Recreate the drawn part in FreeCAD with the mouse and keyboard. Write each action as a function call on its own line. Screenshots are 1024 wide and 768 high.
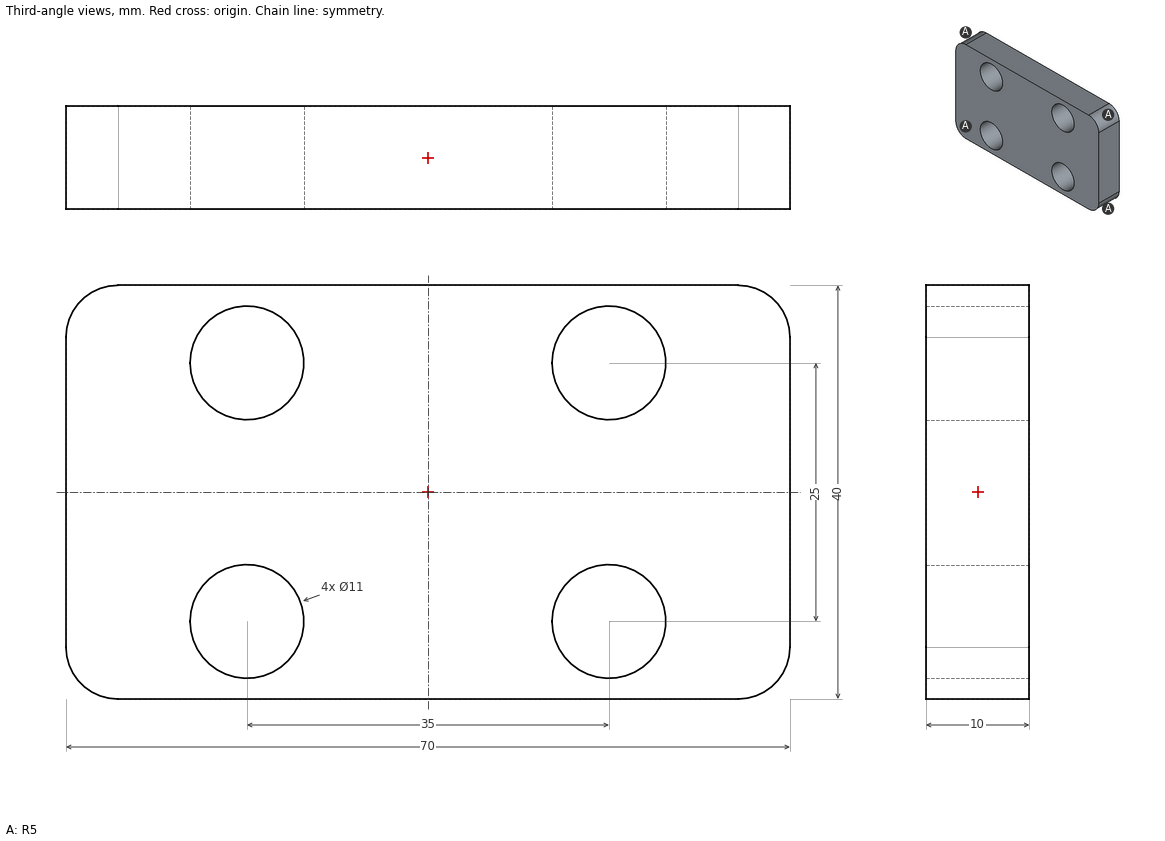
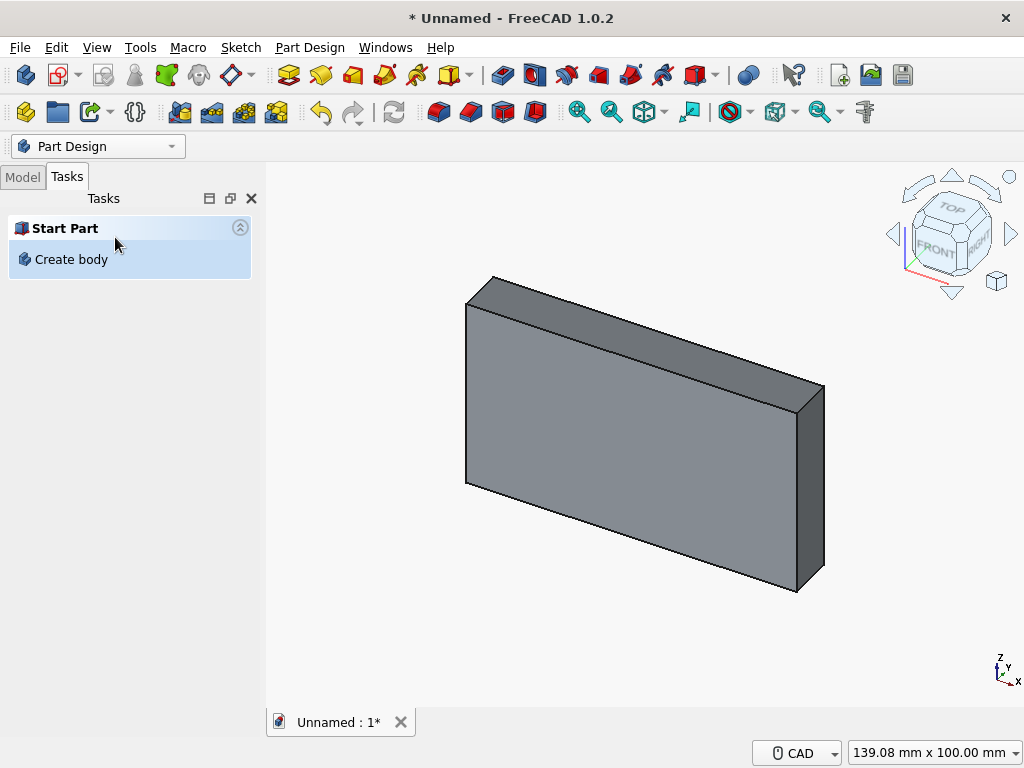
key(4)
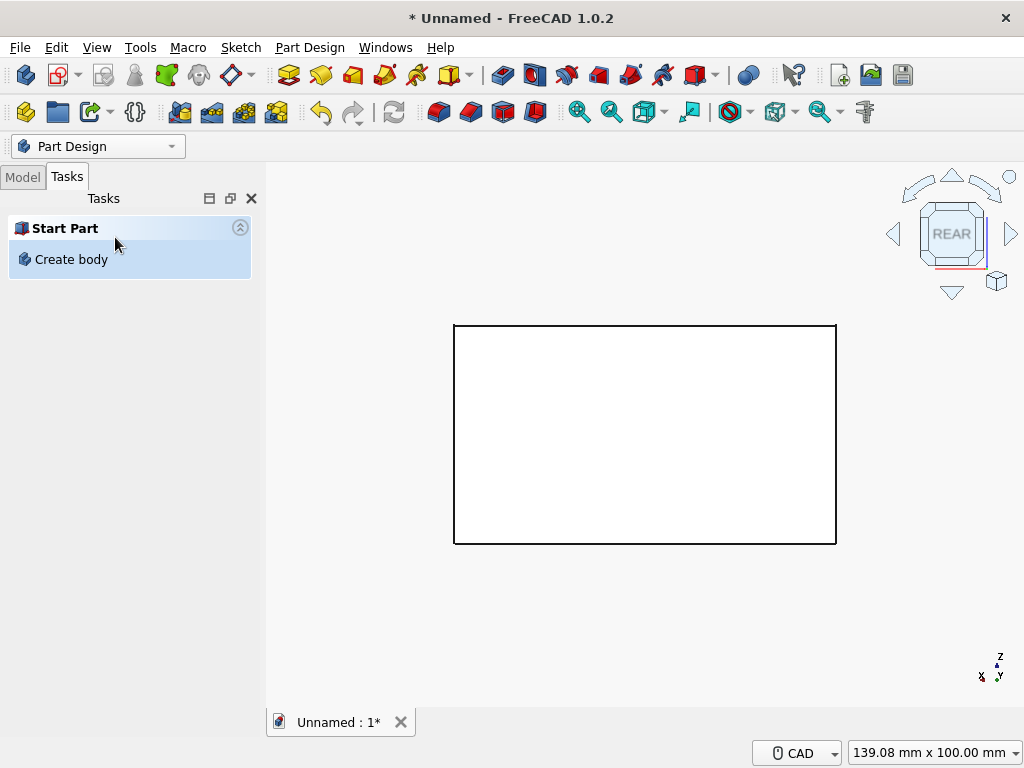
click(591, 433)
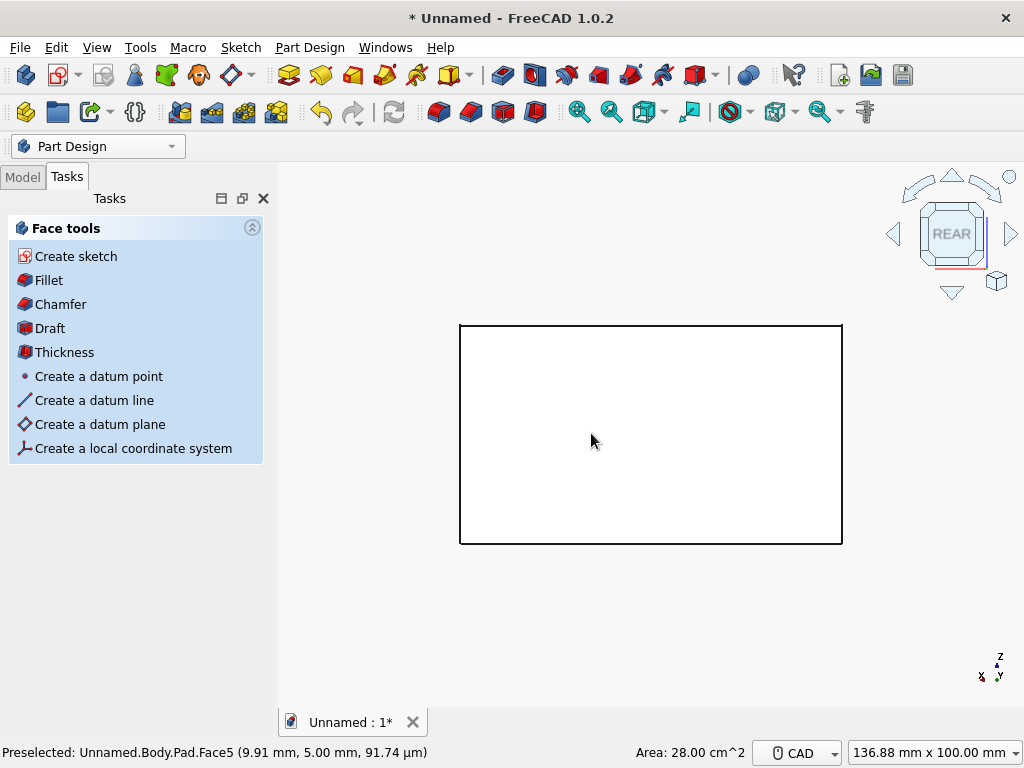
click(58, 76)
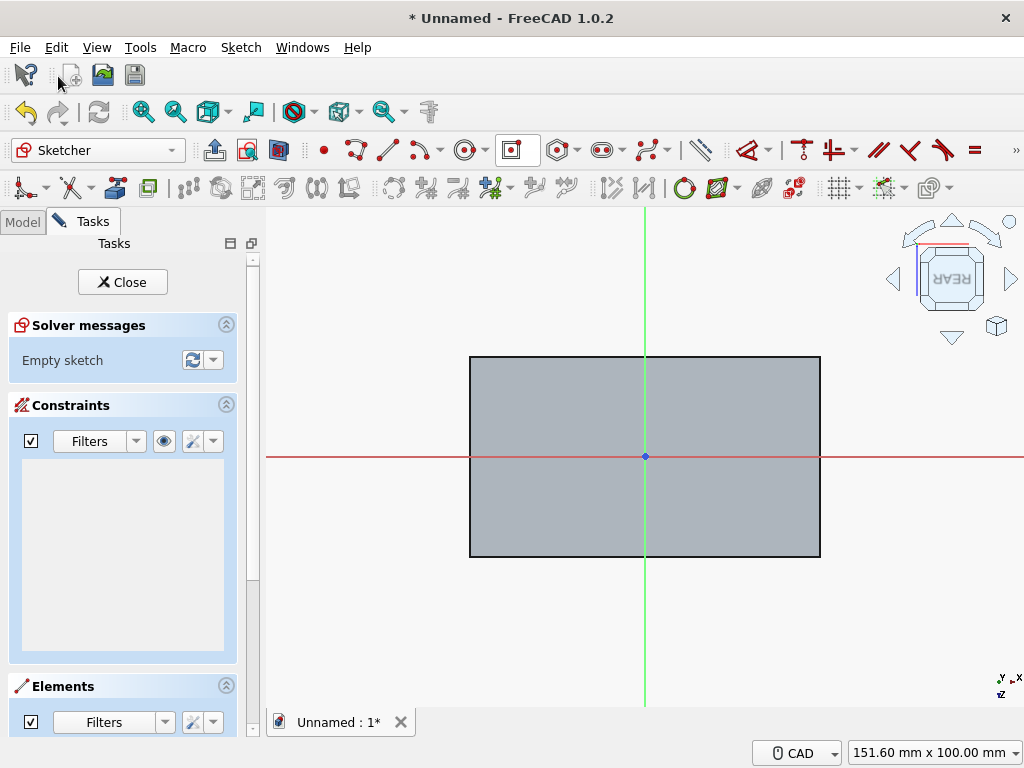
scroll(728, 457, up, 3)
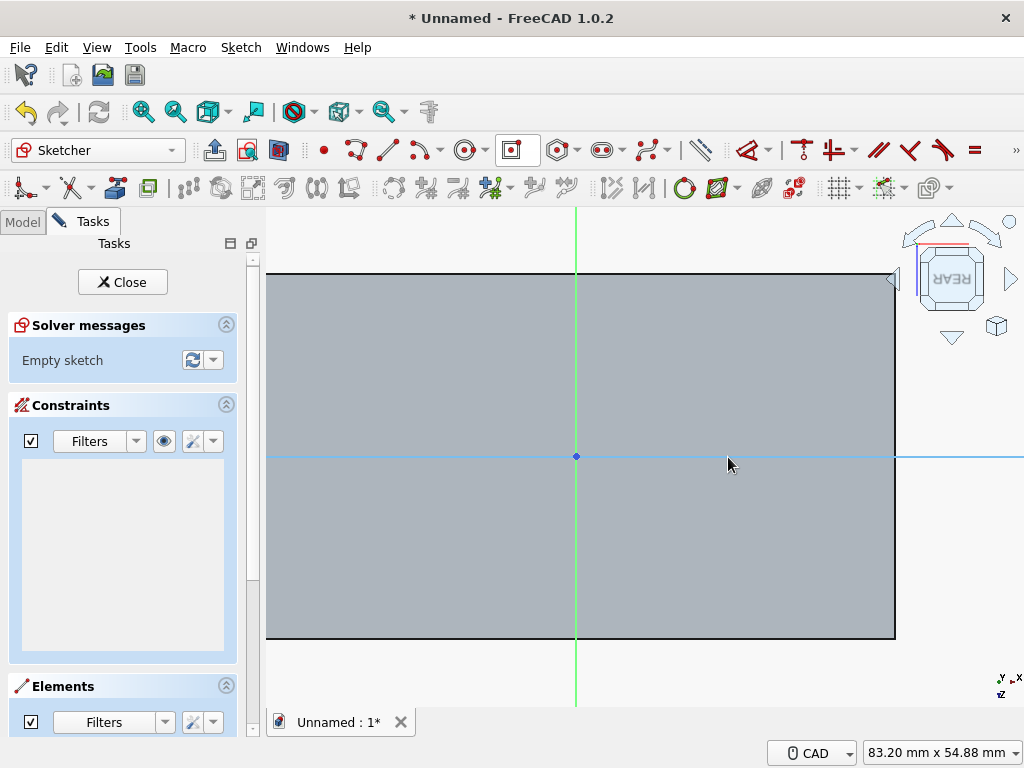
click(466, 150)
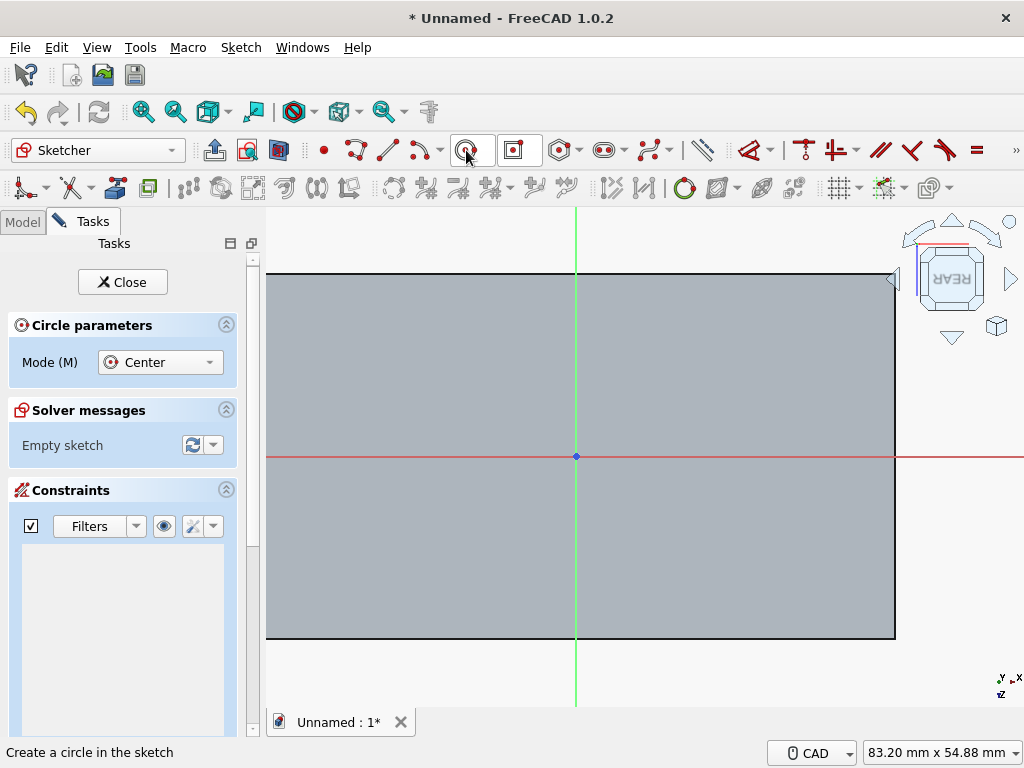
click(417, 343)
move(452, 307)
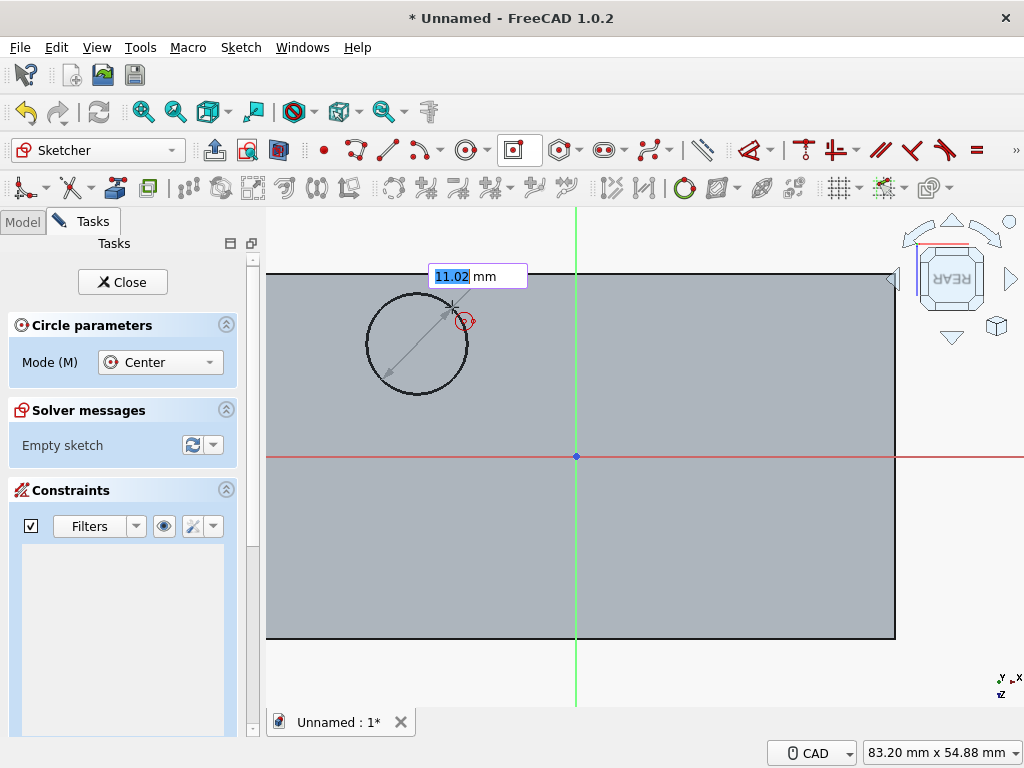
text(11)
key(Return)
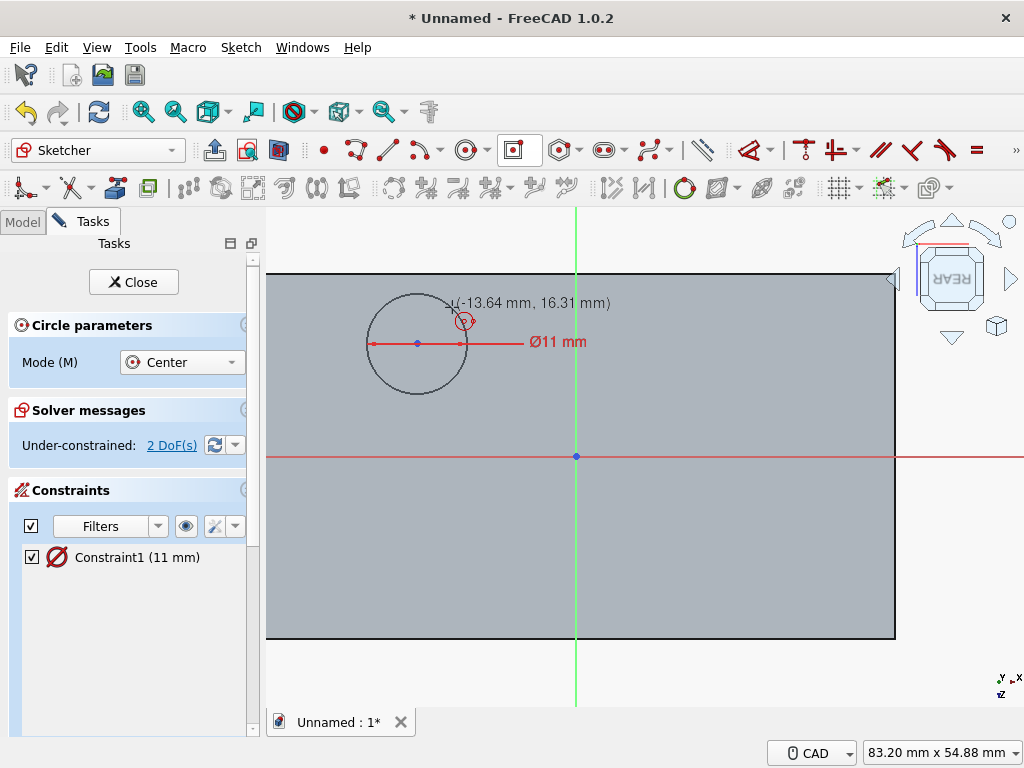
click(736, 343)
move(771, 307)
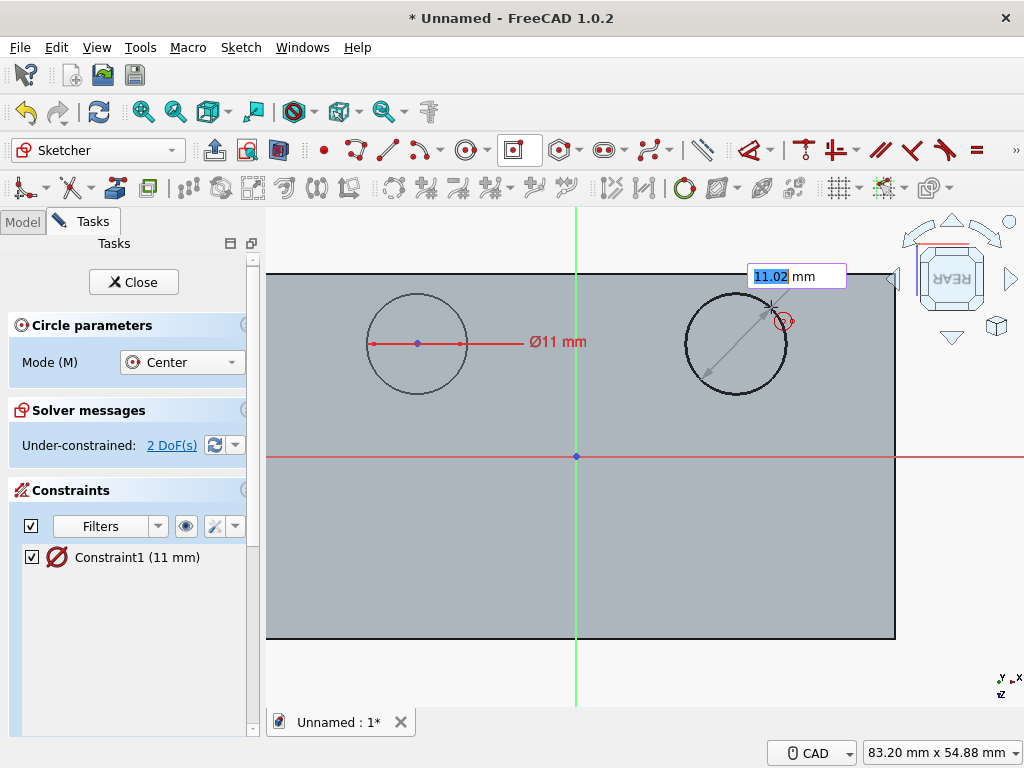
text(11)
key(Return)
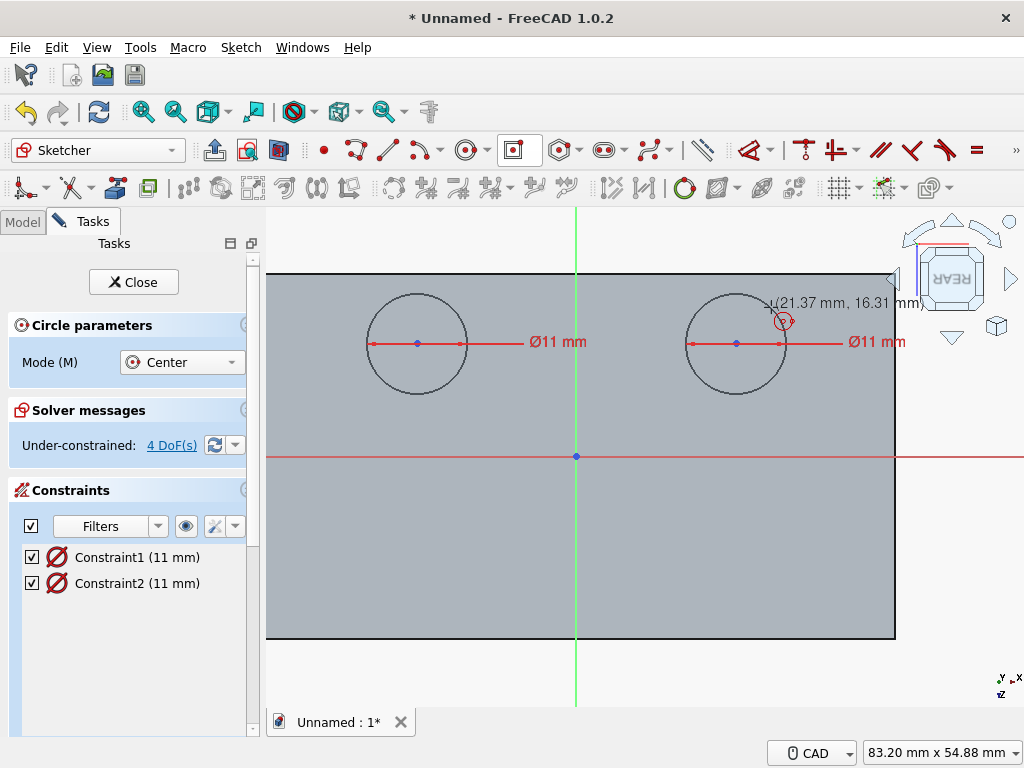
click(736, 570)
move(771, 535)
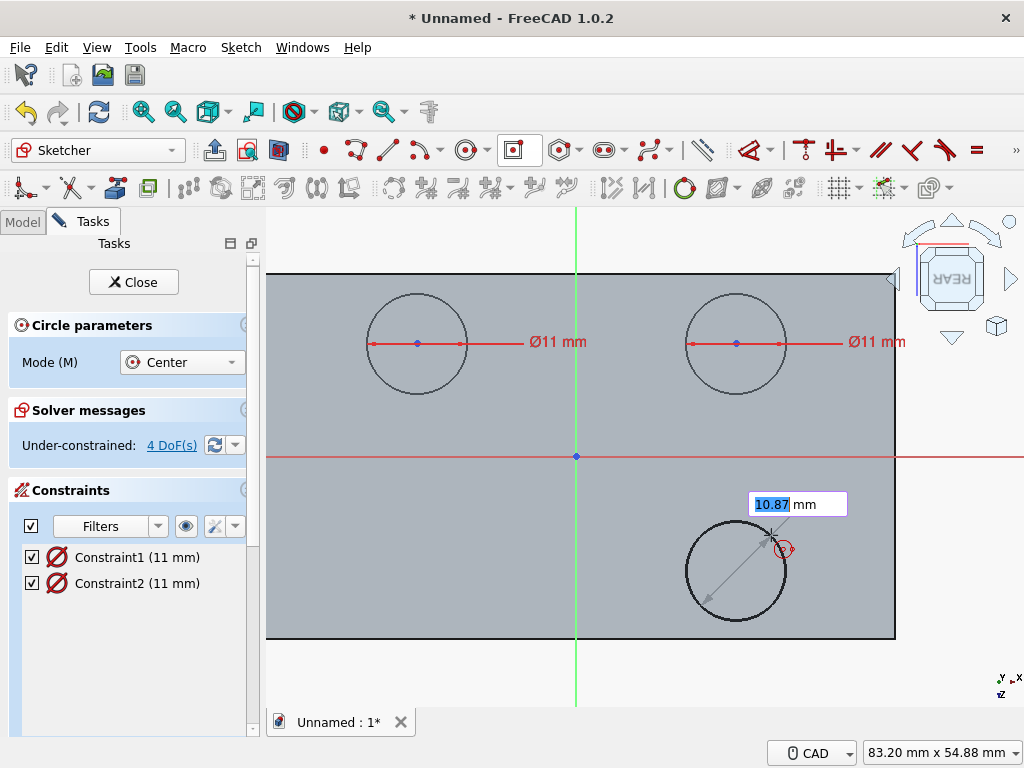
text(11)
key(Return)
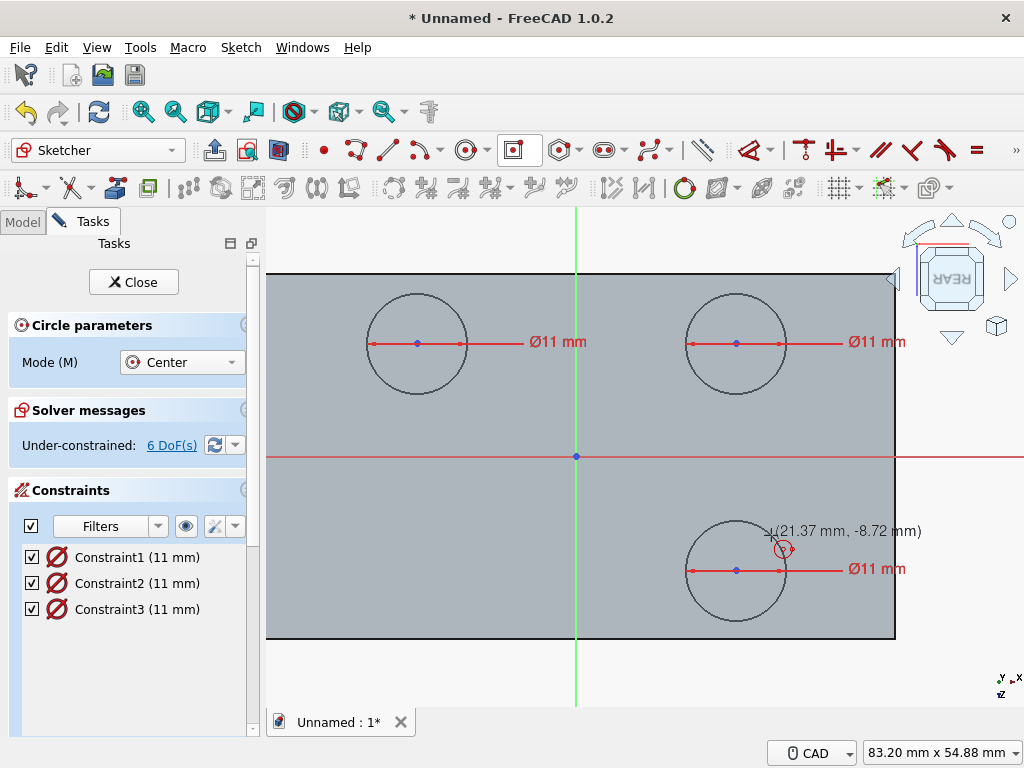
click(417, 570)
move(452, 535)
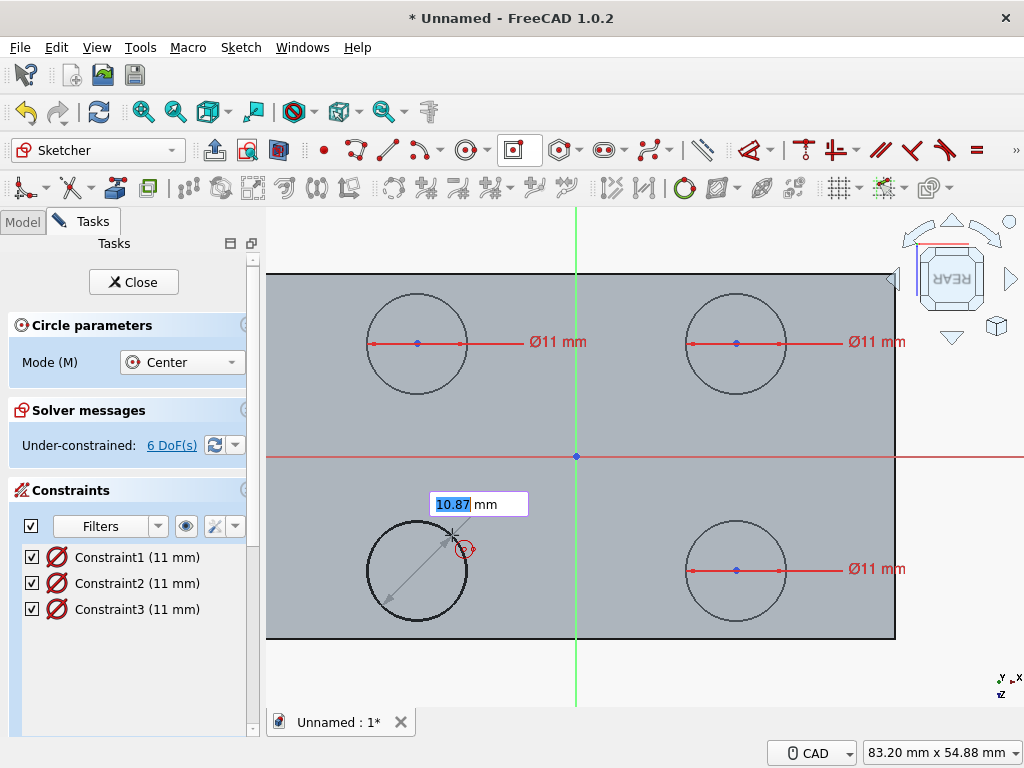
text(11)
key(Return)
key(Escape)